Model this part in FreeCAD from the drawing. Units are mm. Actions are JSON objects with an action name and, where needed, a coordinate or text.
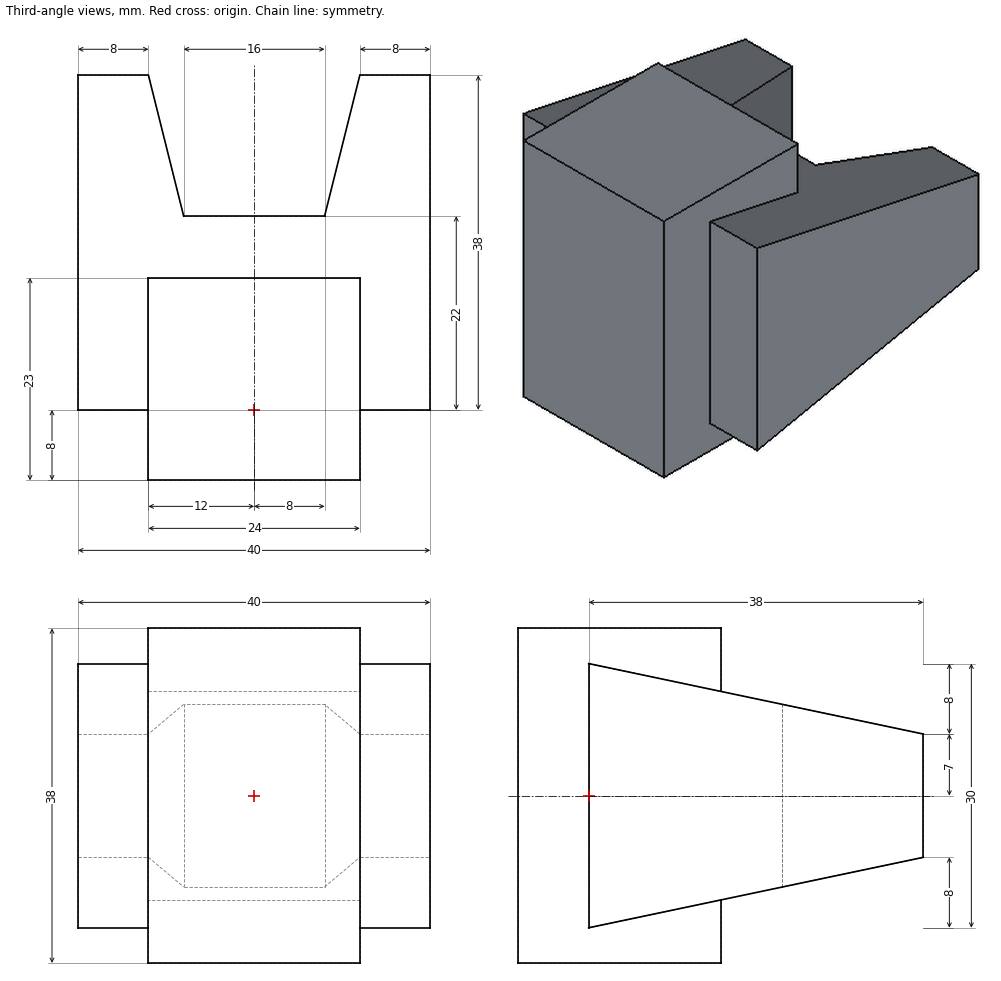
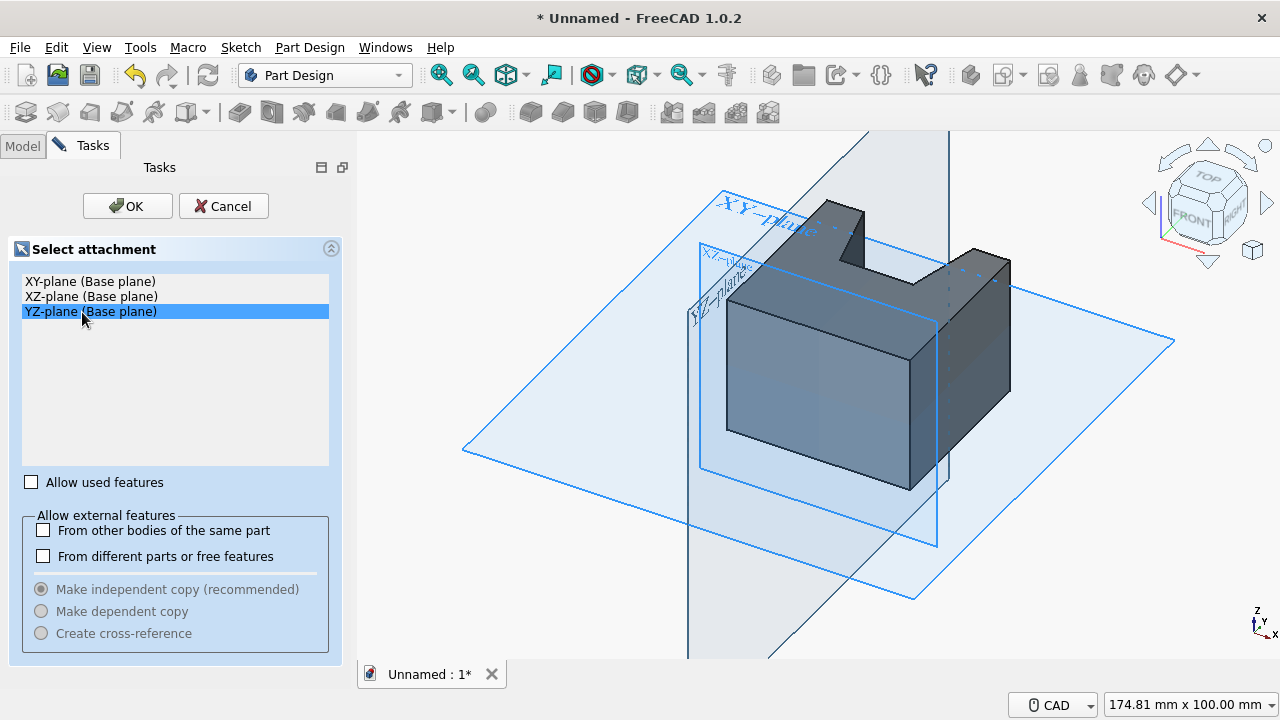
{"action": "left_click", "coordinate": [128, 206]}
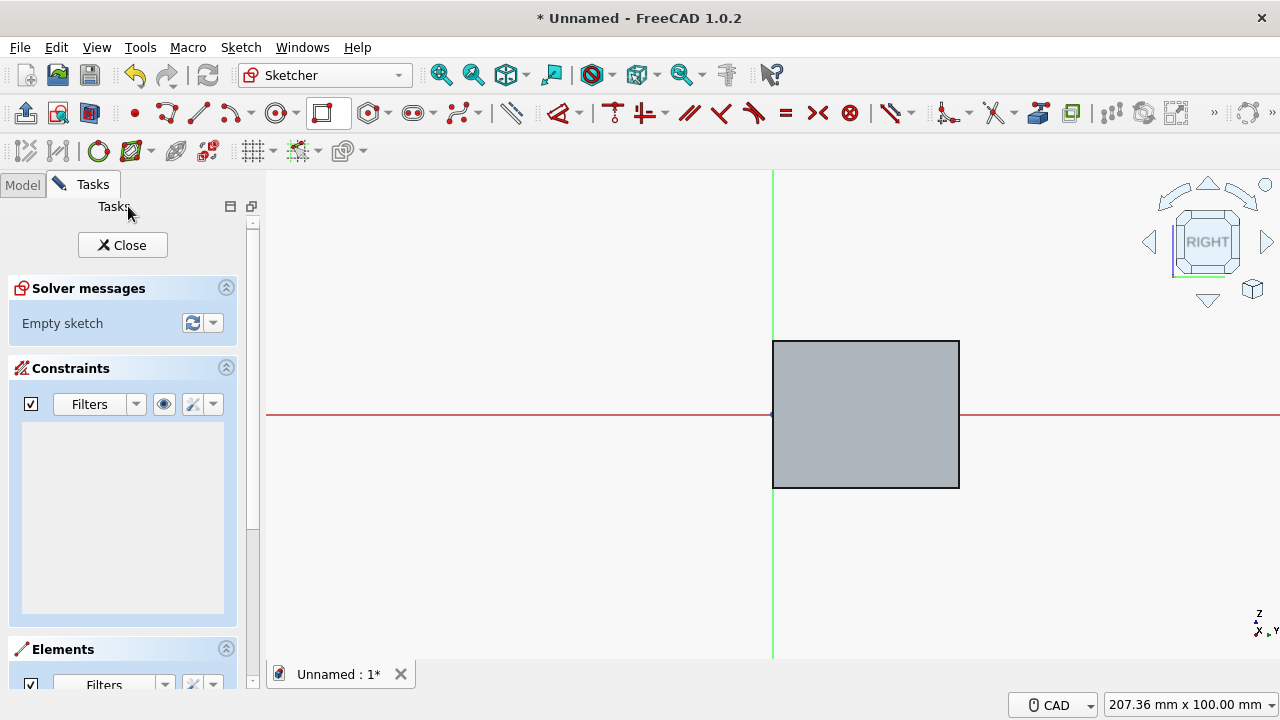
{"action": "left_click", "coordinate": [90, 114]}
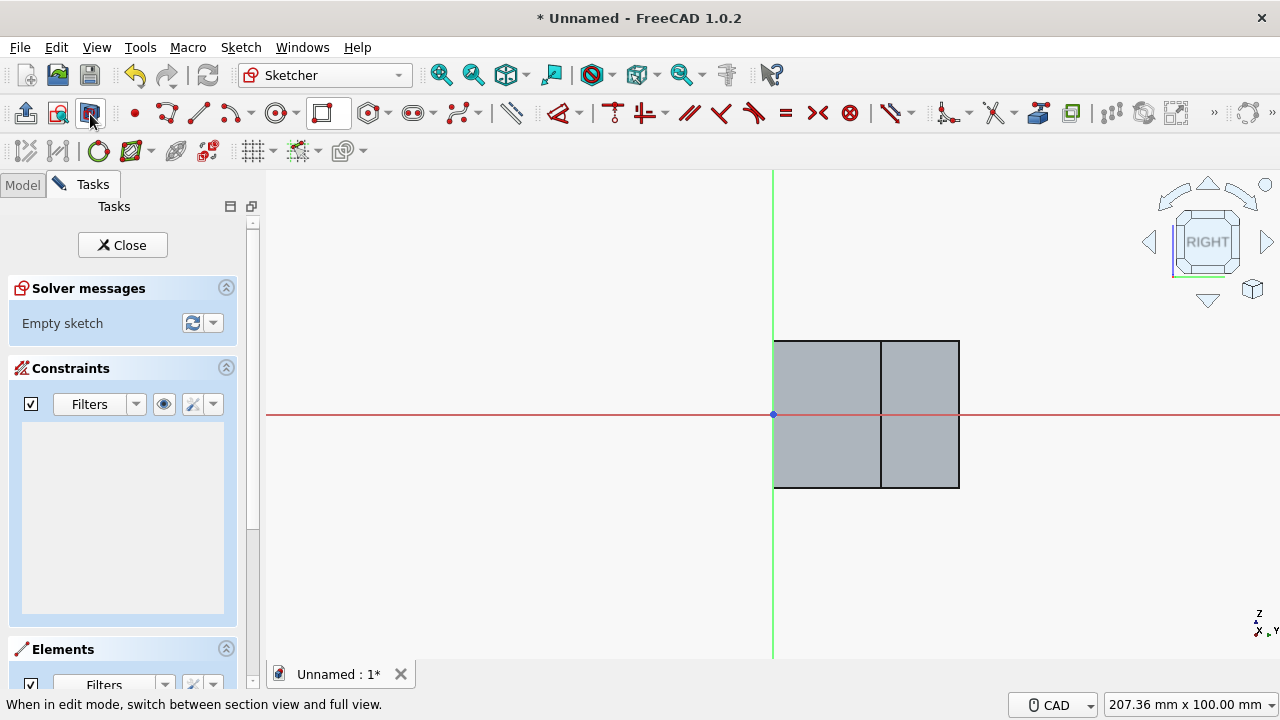
{"action": "scroll", "coordinate": [998, 414], "scroll_direction": "up", "scroll_amount": 4}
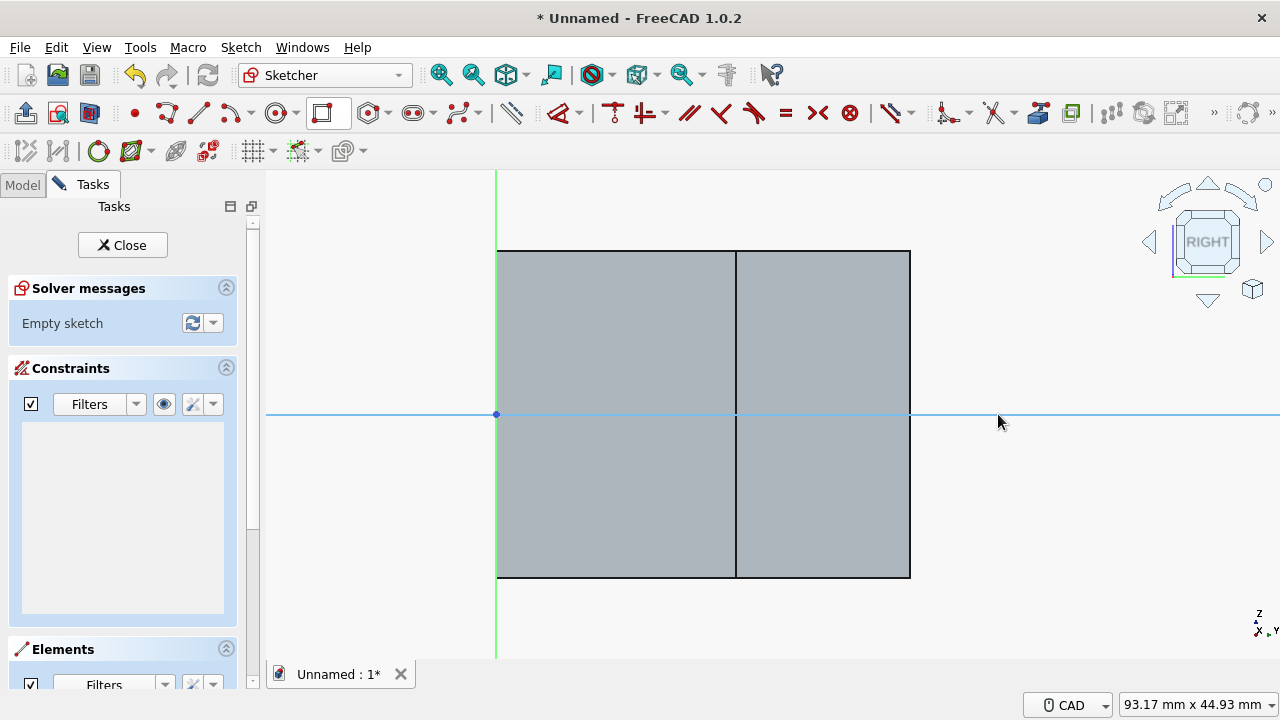
{"action": "left_click", "coordinate": [168, 114]}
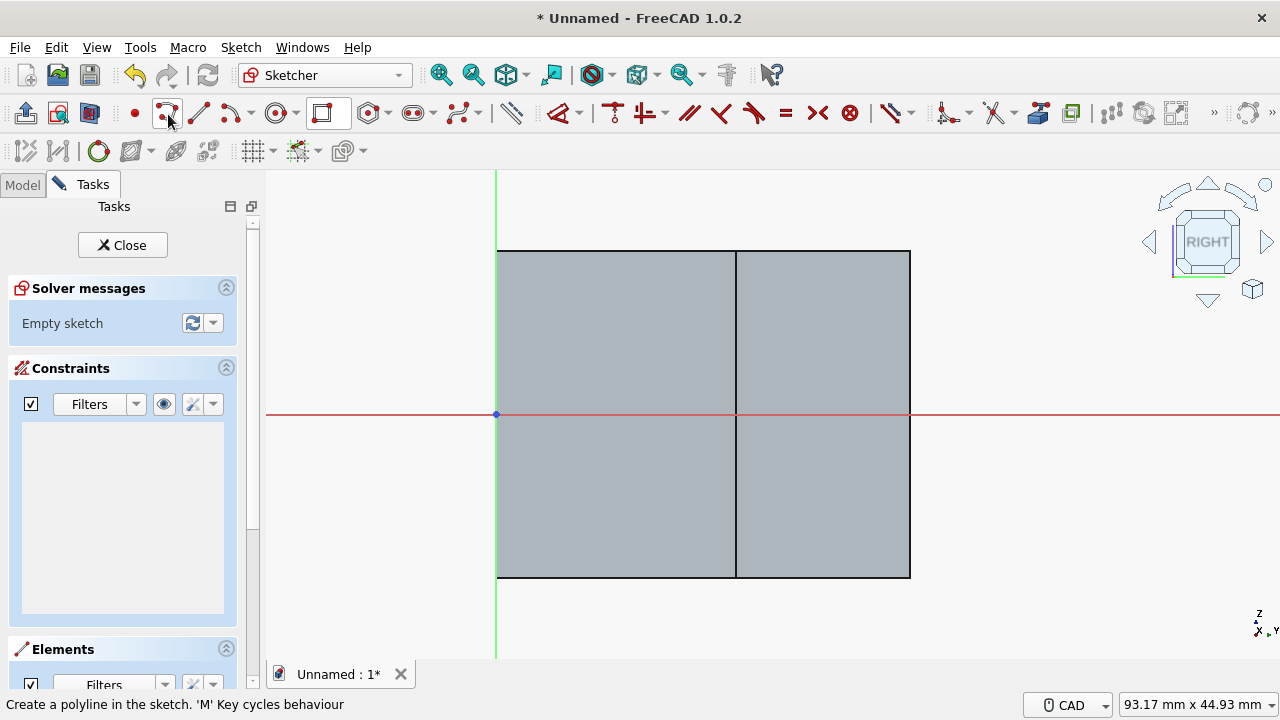
{"action": "left_click", "coordinate": [496, 251]}
{"action": "left_click", "coordinate": [910, 338]}
{"action": "left_click", "coordinate": [910, 251]}
{"action": "left_click", "coordinate": [496, 252]}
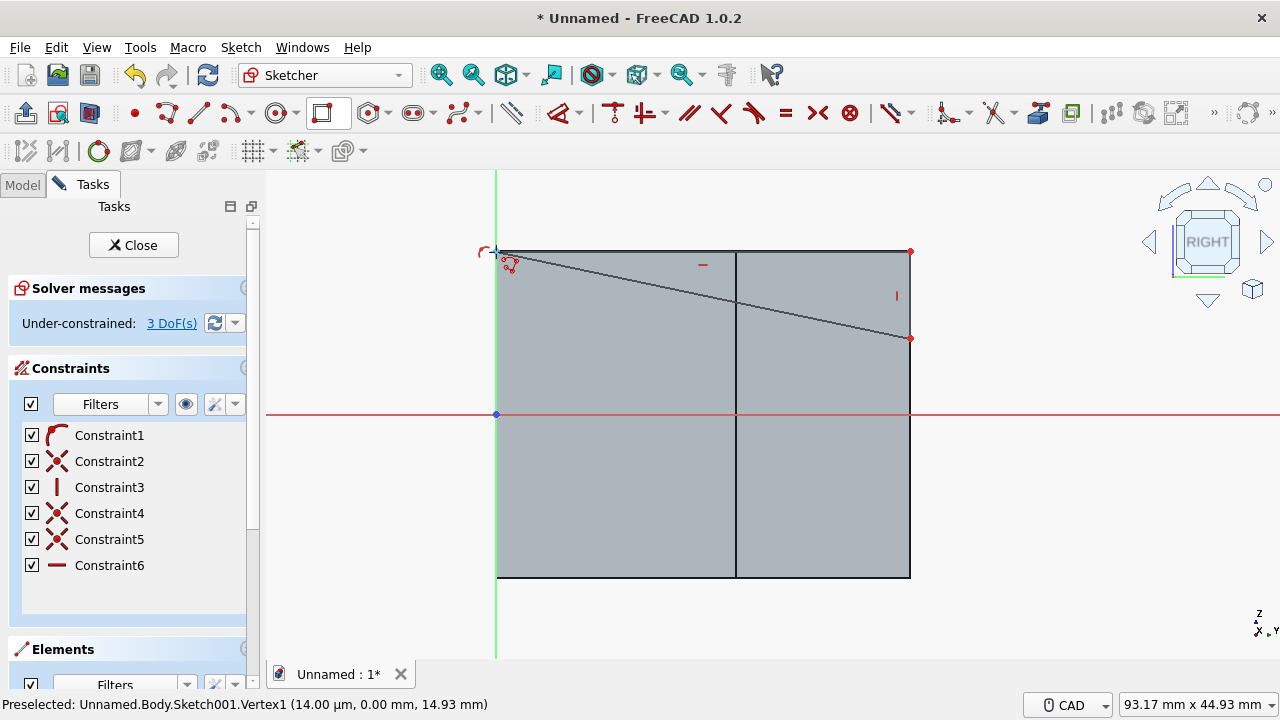
{"action": "left_click", "coordinate": [496, 578]}
{"action": "left_click", "coordinate": [910, 578]}
{"action": "left_click", "coordinate": [910, 491]}
{"action": "left_click", "coordinate": [496, 579]}
{"action": "key", "text": "Escape"}
{"action": "key", "text": "Escape"}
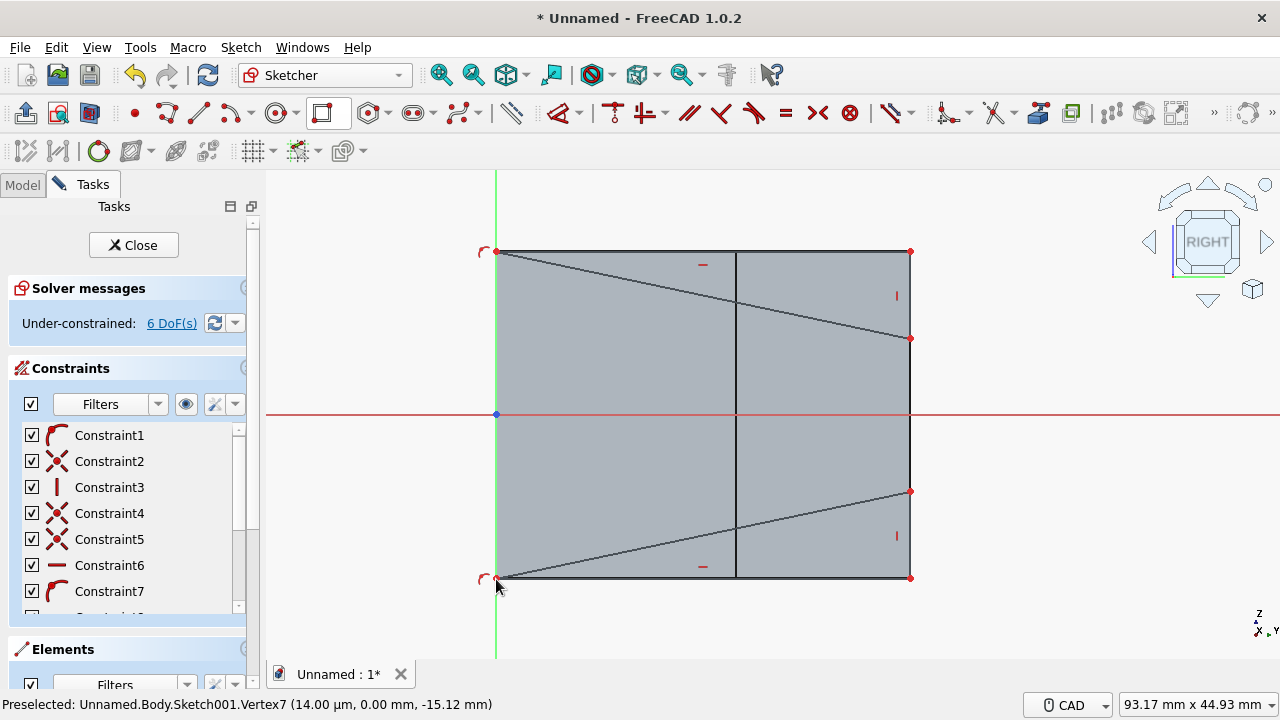
{"action": "left_click", "coordinate": [910, 252]}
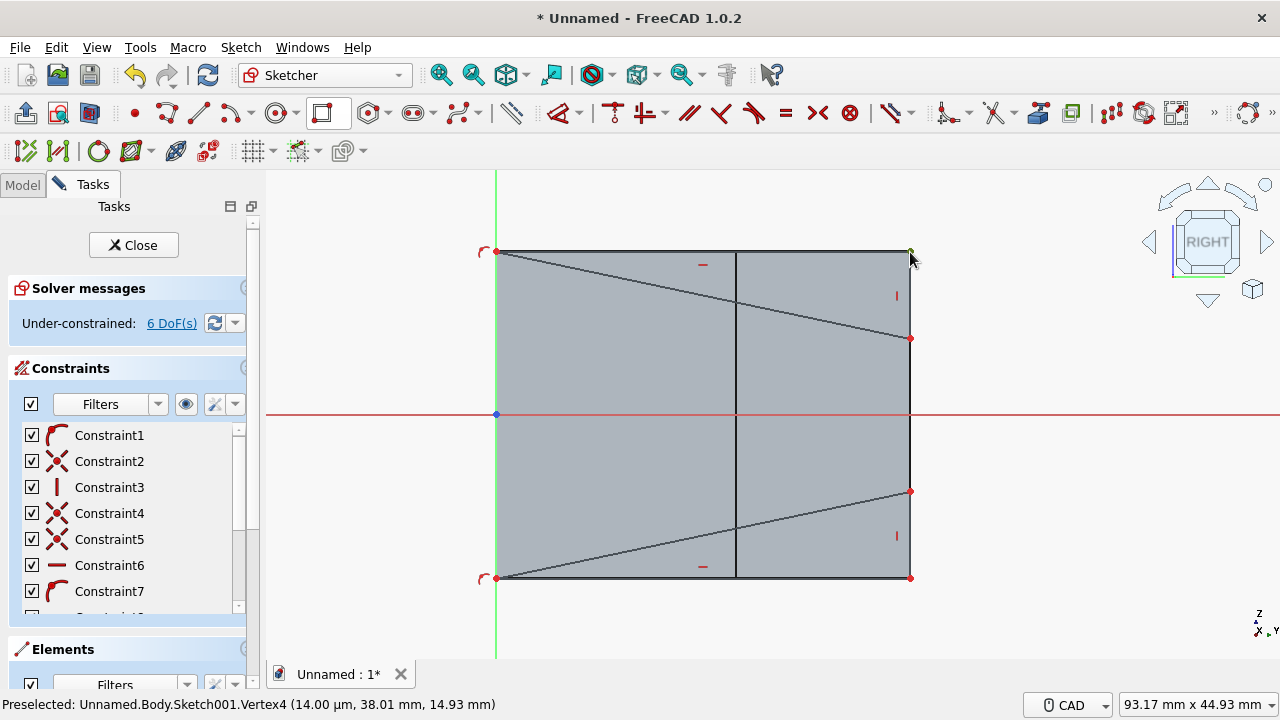
{"action": "left_click", "coordinate": [910, 579]}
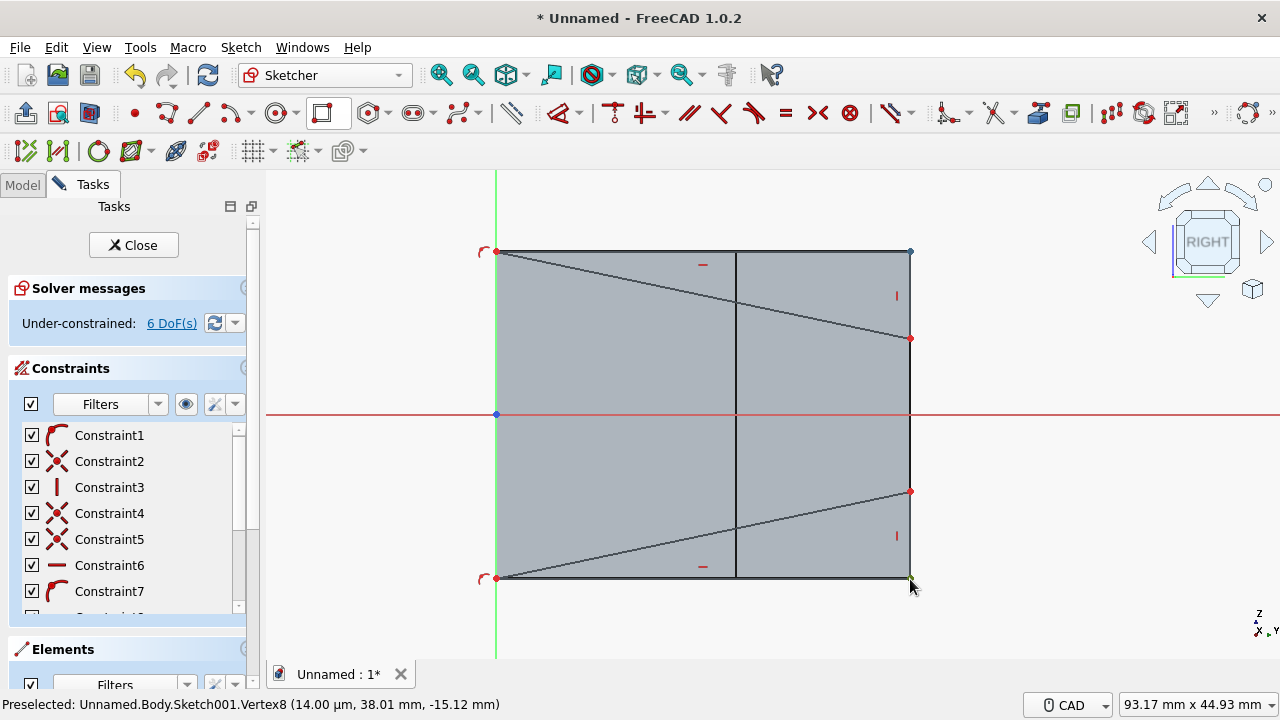
{"action": "left_click", "coordinate": [353, 414]}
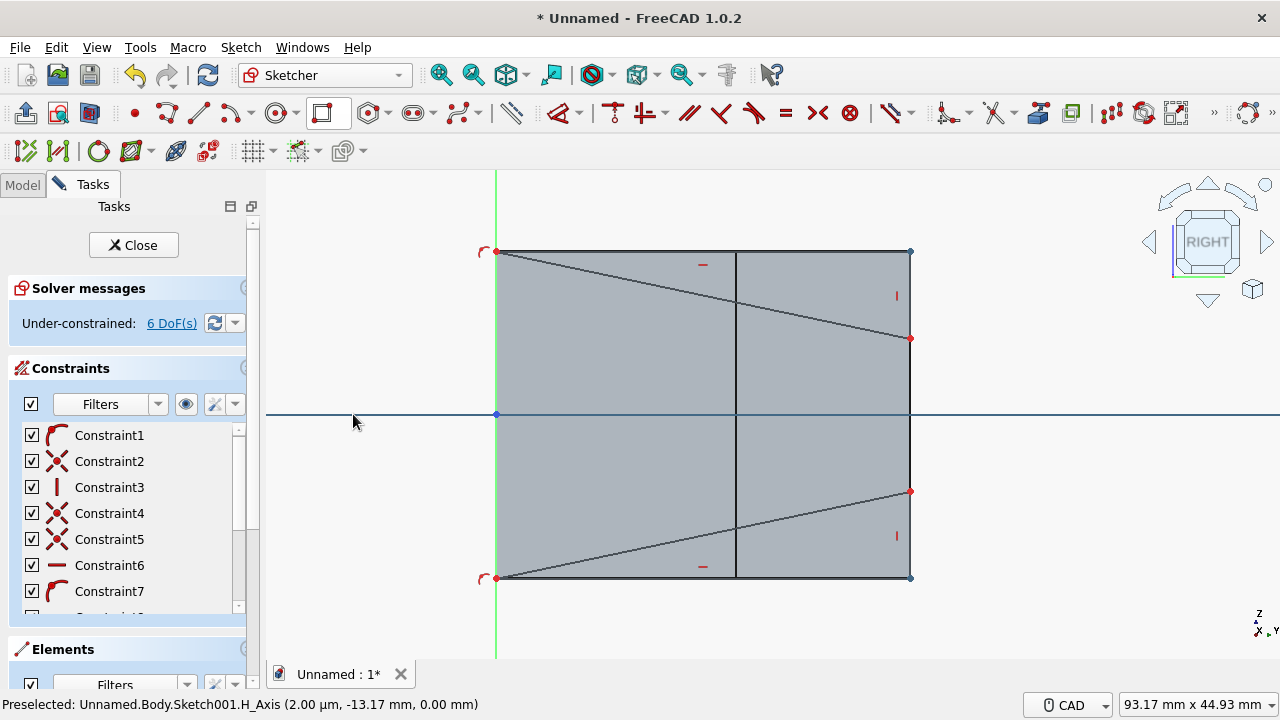
{"action": "left_click", "coordinate": [818, 114]}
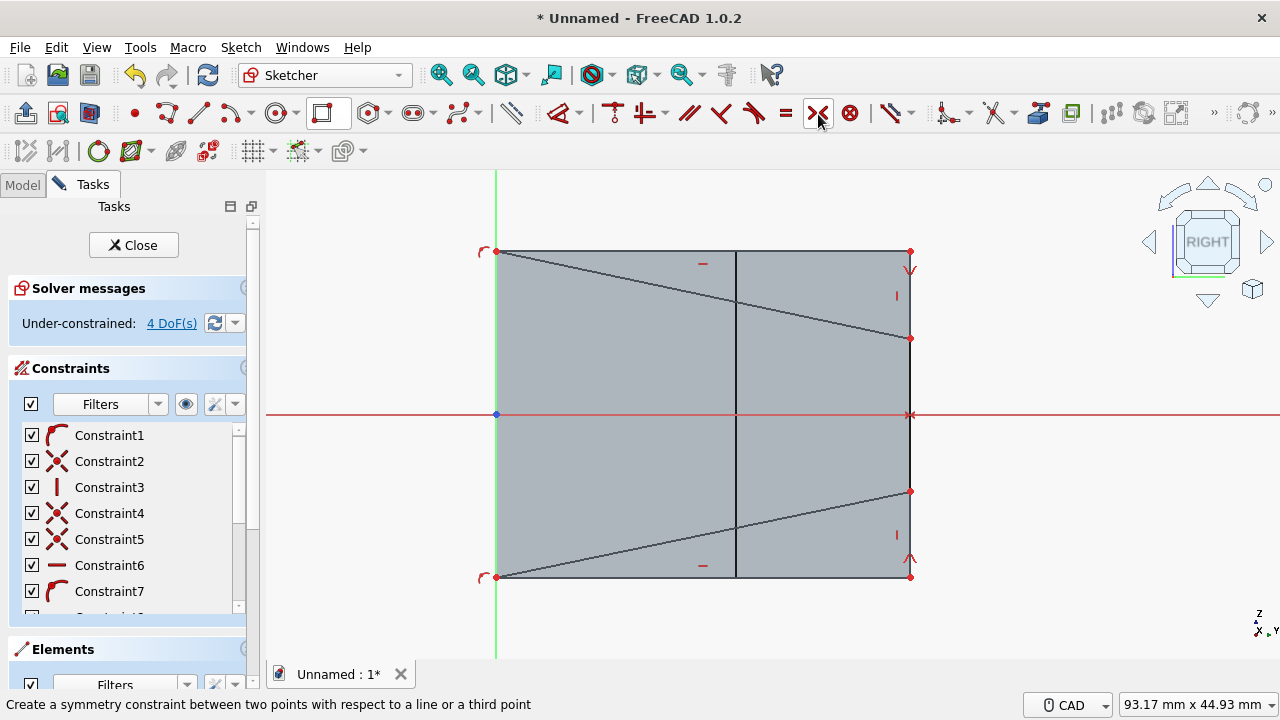
{"action": "left_click", "coordinate": [558, 114]}